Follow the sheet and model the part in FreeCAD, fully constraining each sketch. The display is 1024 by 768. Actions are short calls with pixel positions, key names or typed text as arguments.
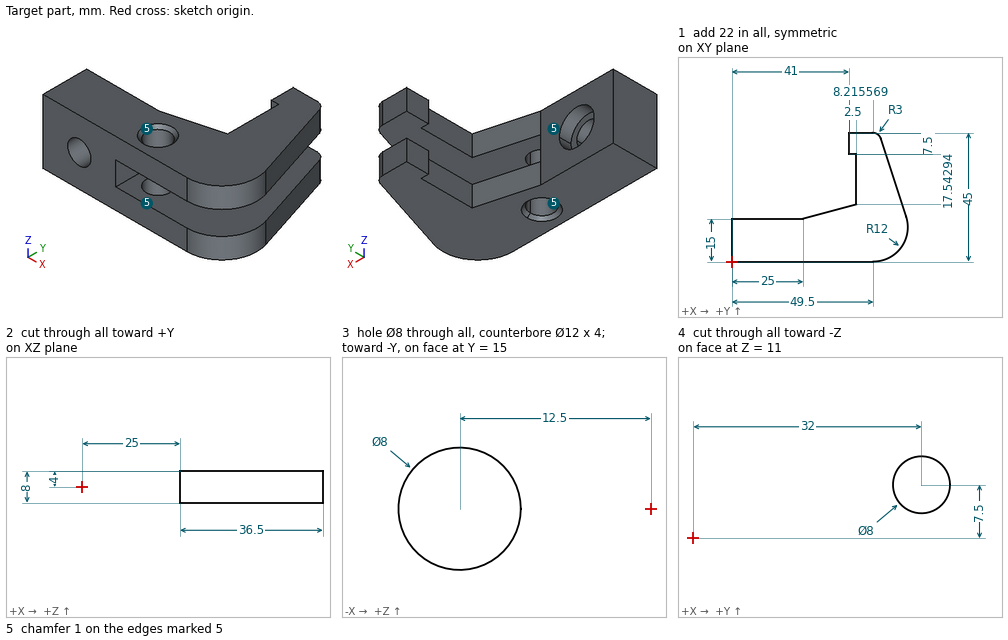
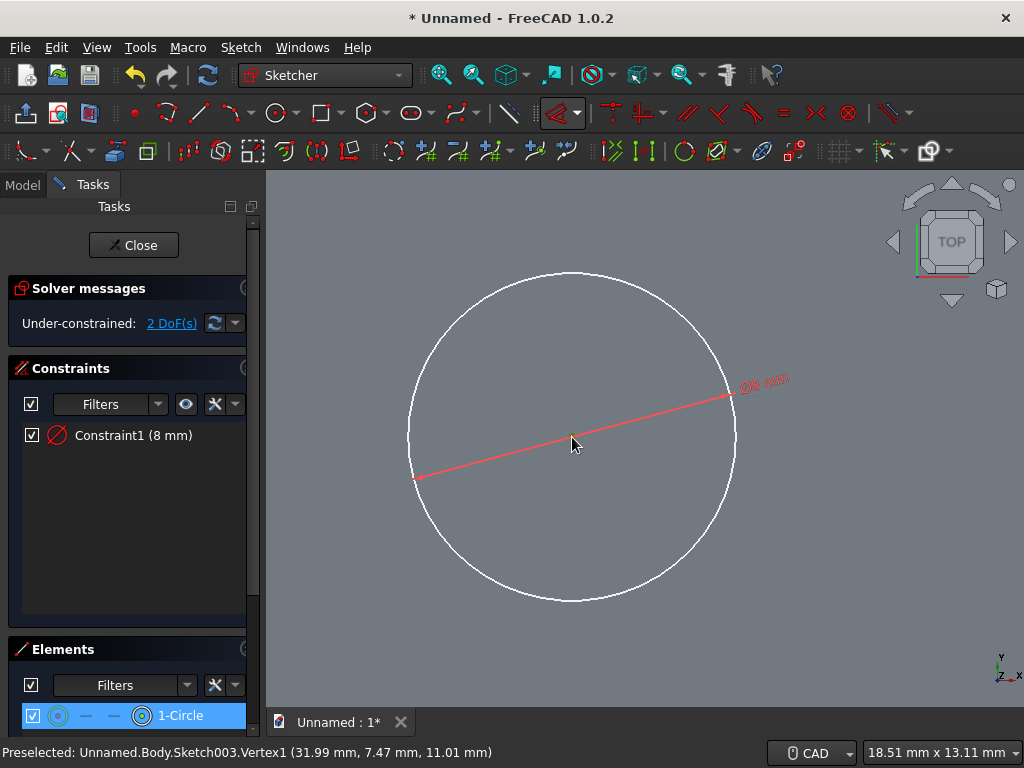
click(580, 114)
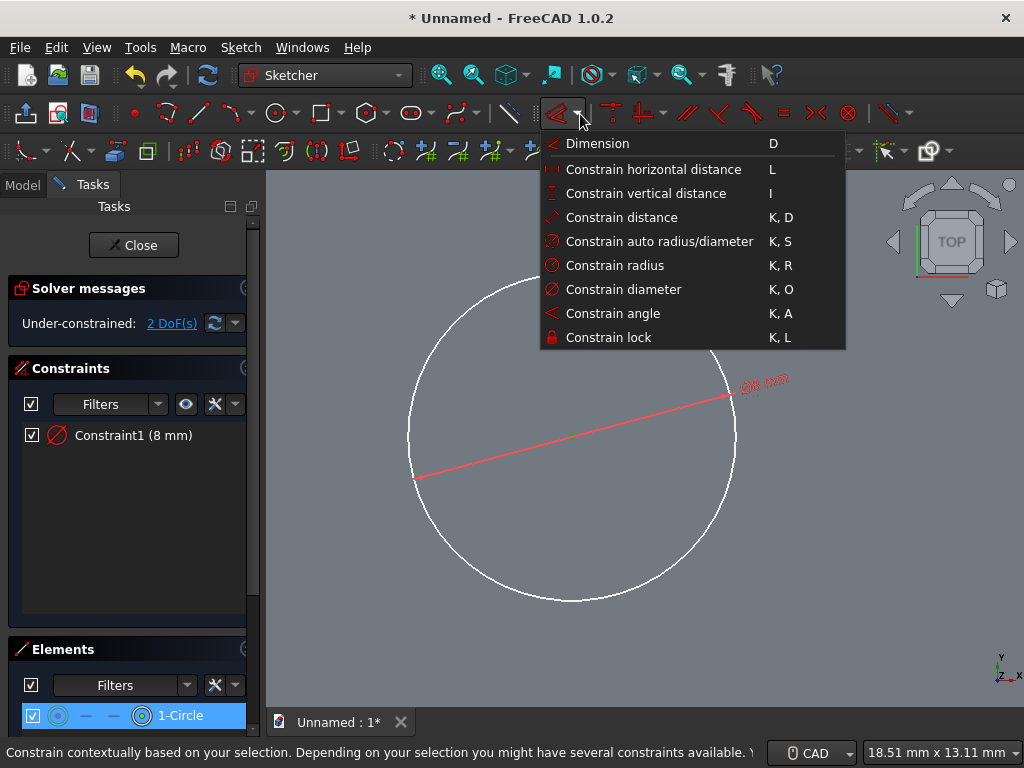
click(693, 169)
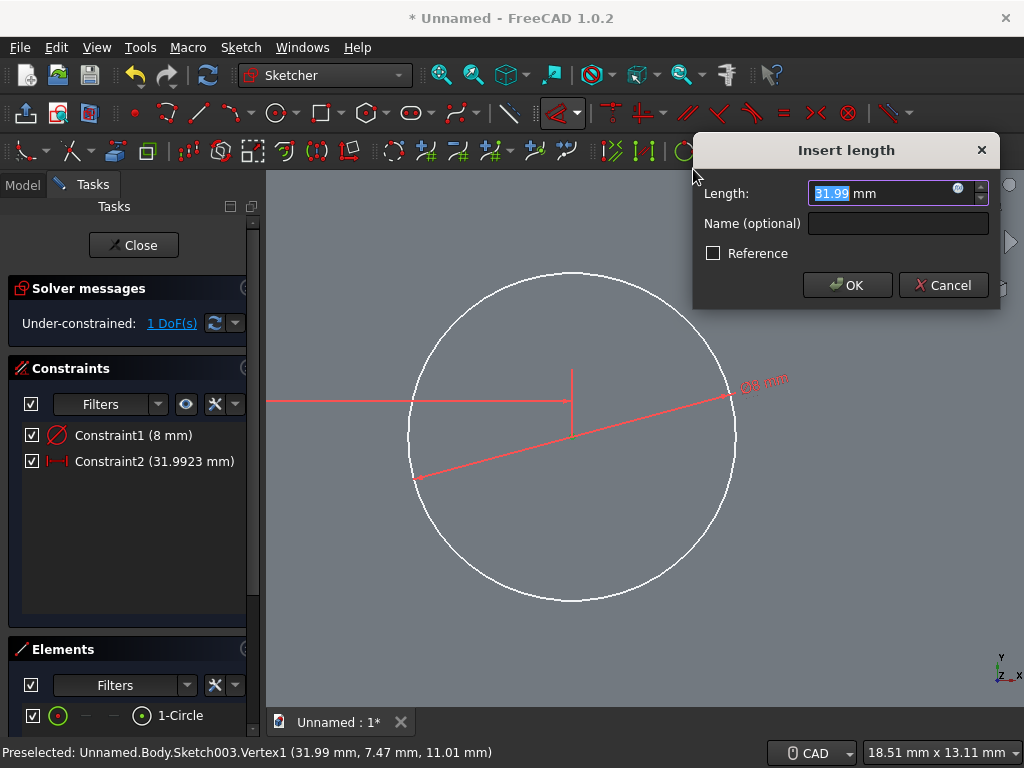
text(32)
key(Return)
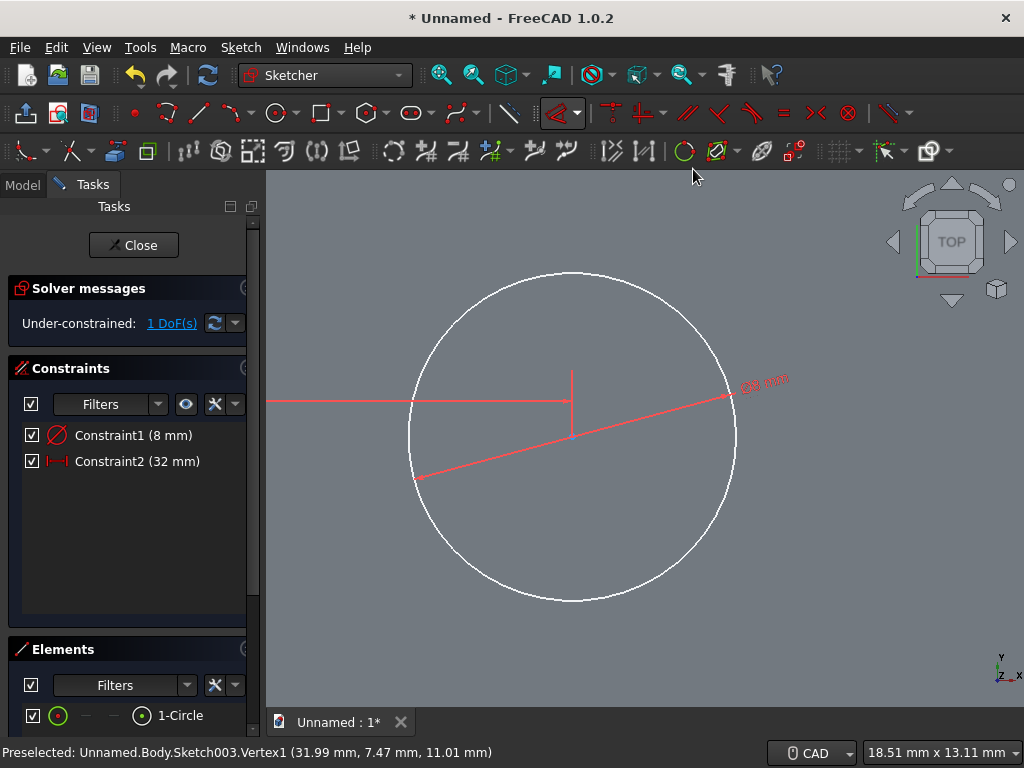
click(572, 437)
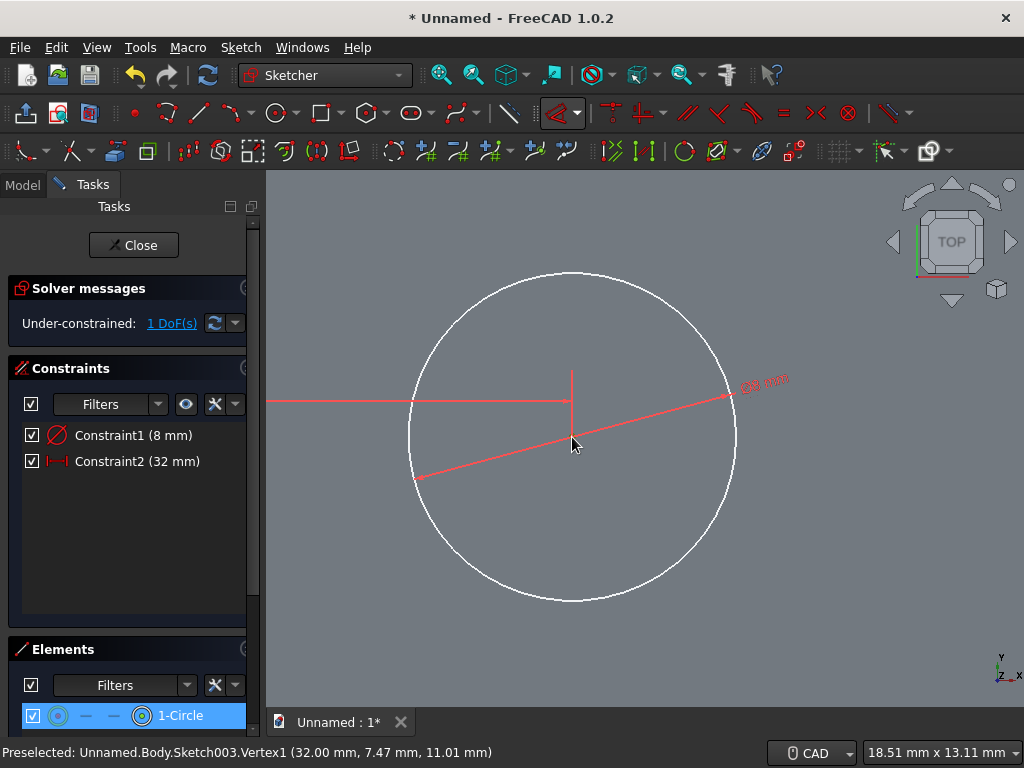
click(580, 114)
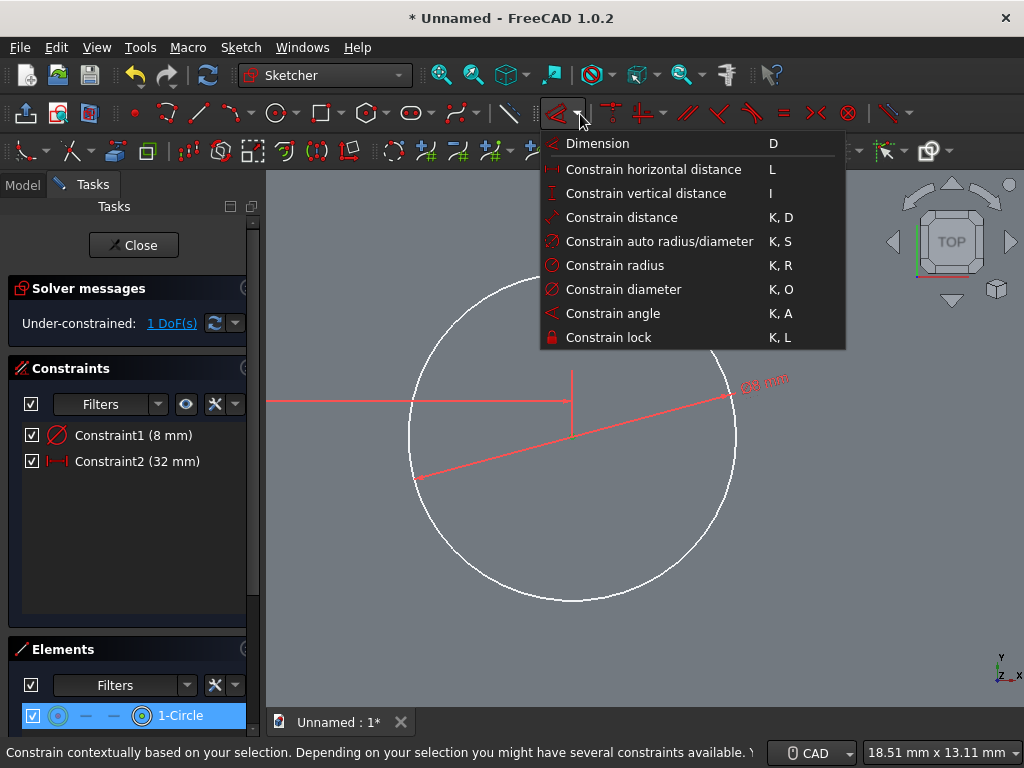
click(693, 193)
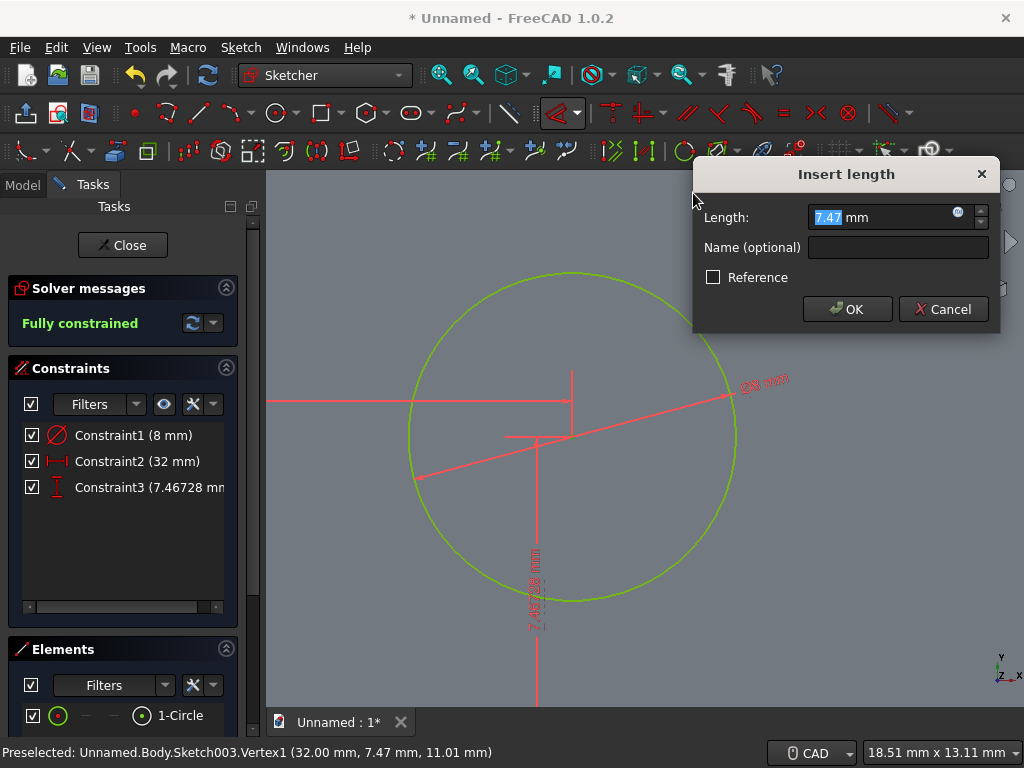
text(7.5)
key(Return)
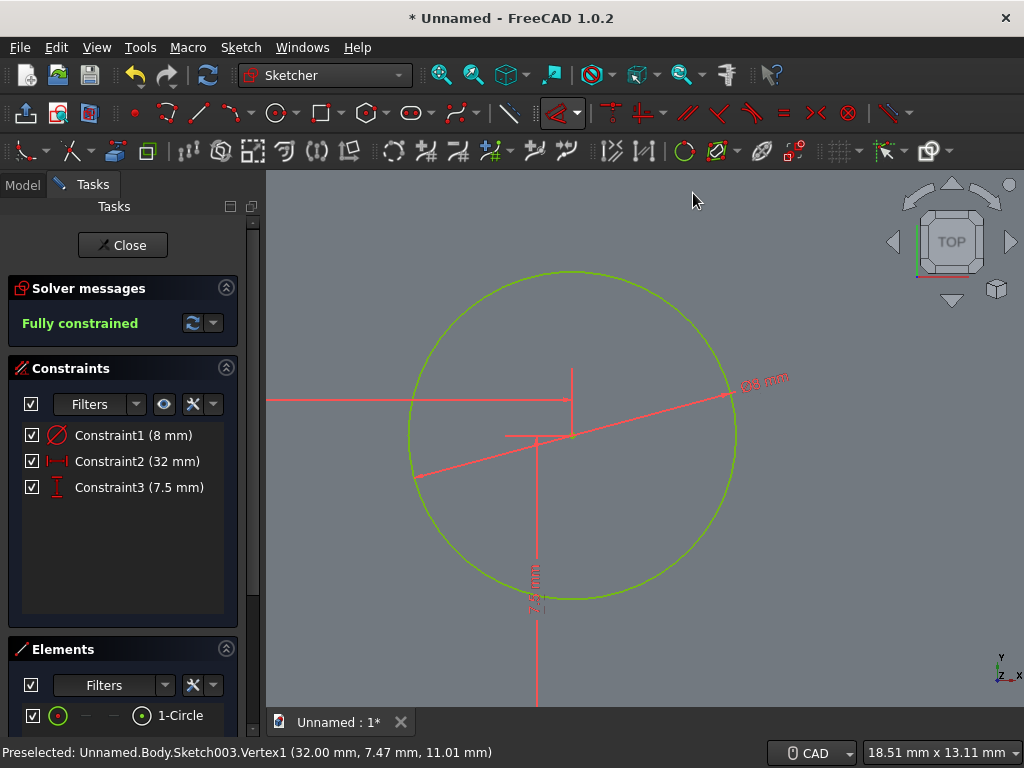
click(123, 245)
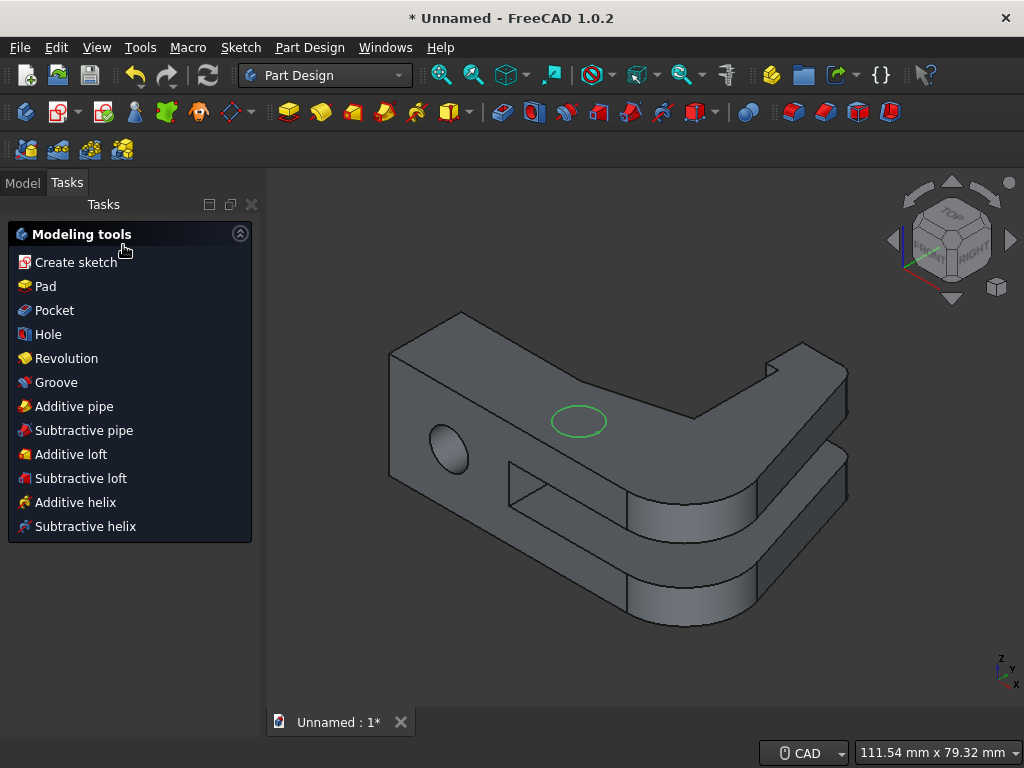
click(504, 112)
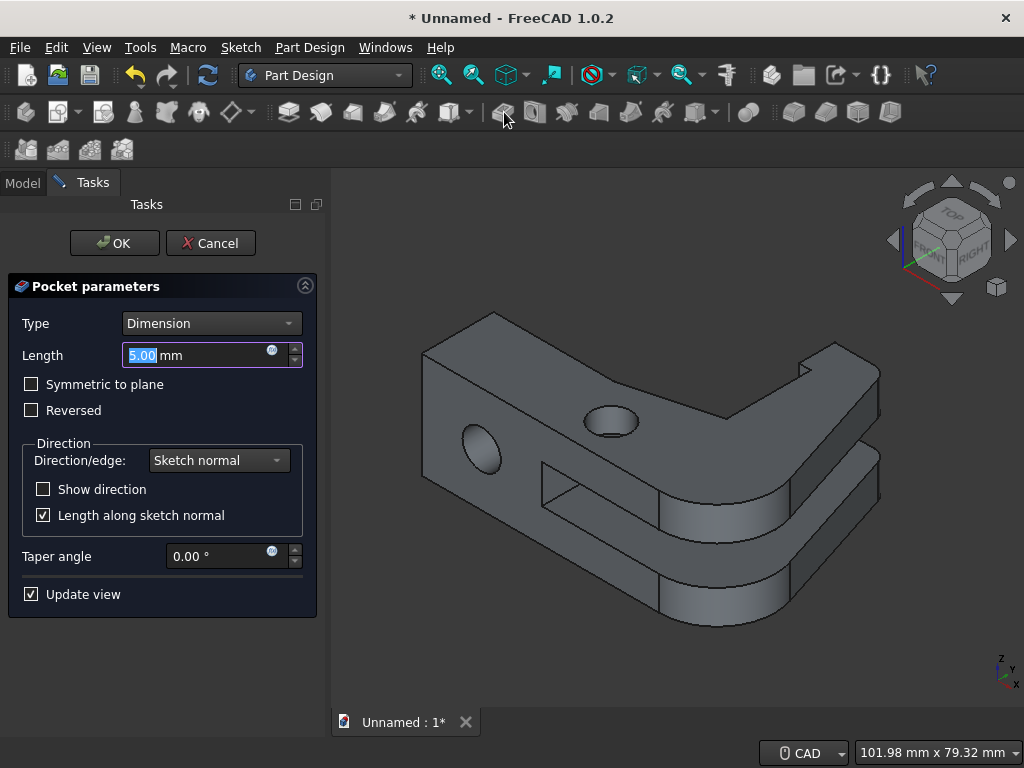
click(212, 324)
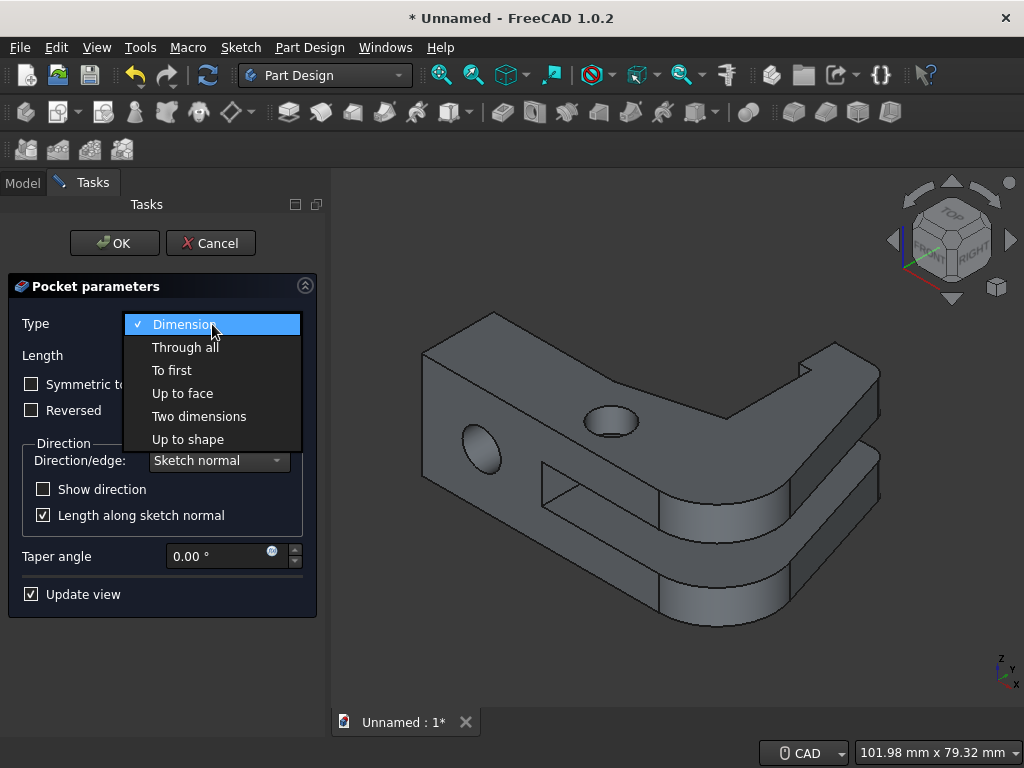
click(212, 348)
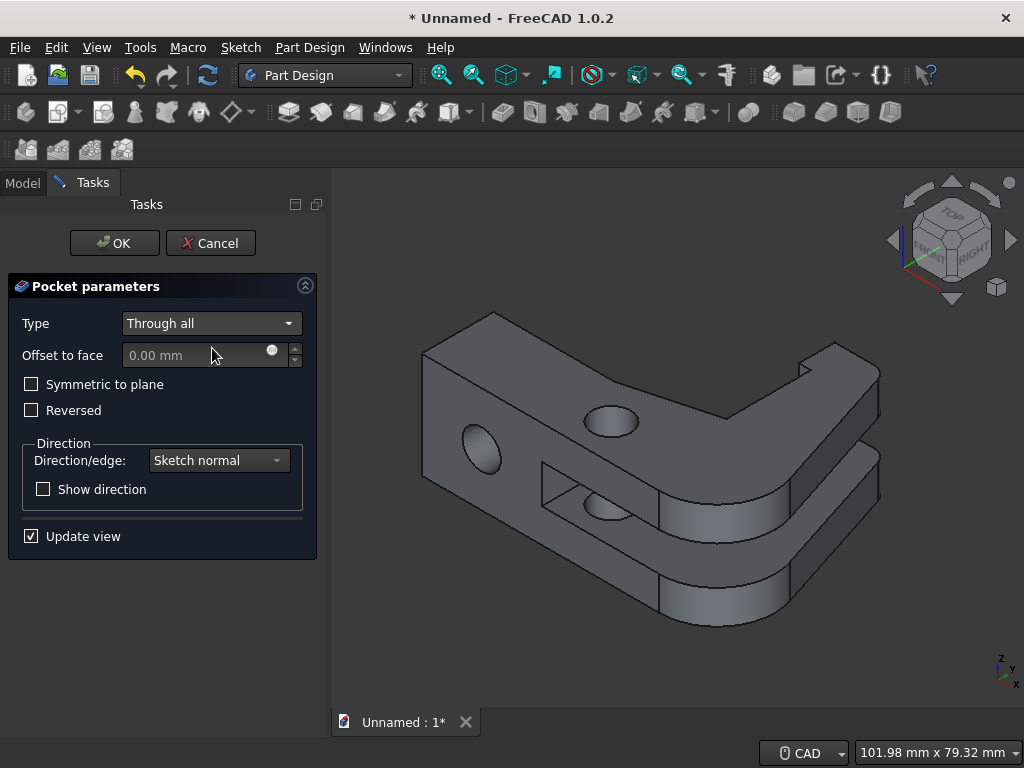
click(115, 243)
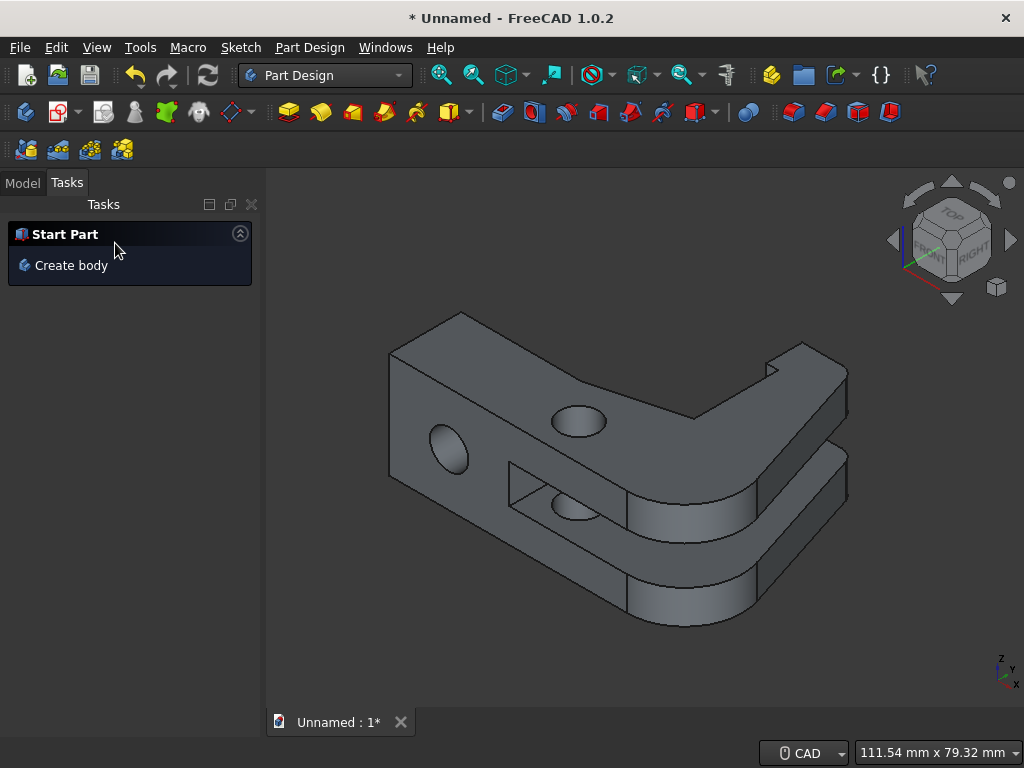
click(560, 409)